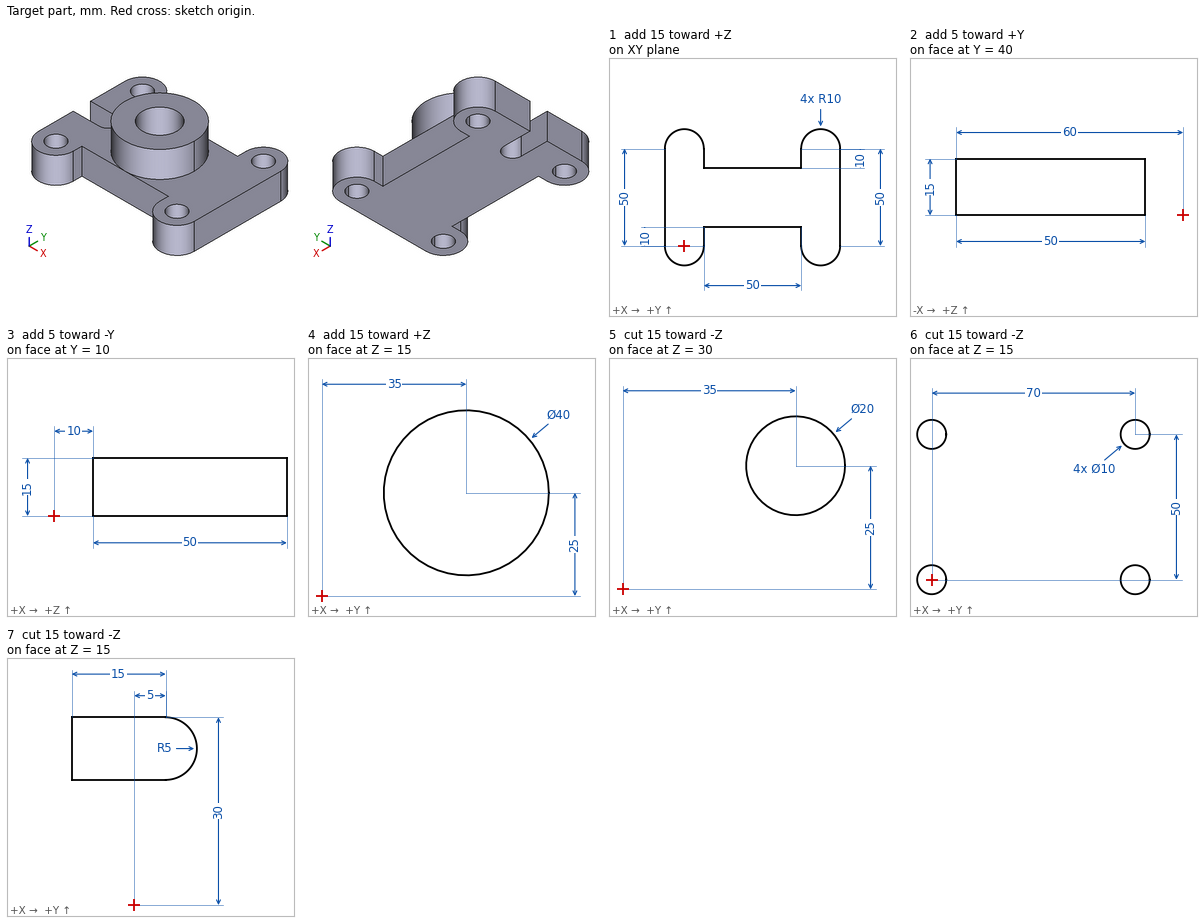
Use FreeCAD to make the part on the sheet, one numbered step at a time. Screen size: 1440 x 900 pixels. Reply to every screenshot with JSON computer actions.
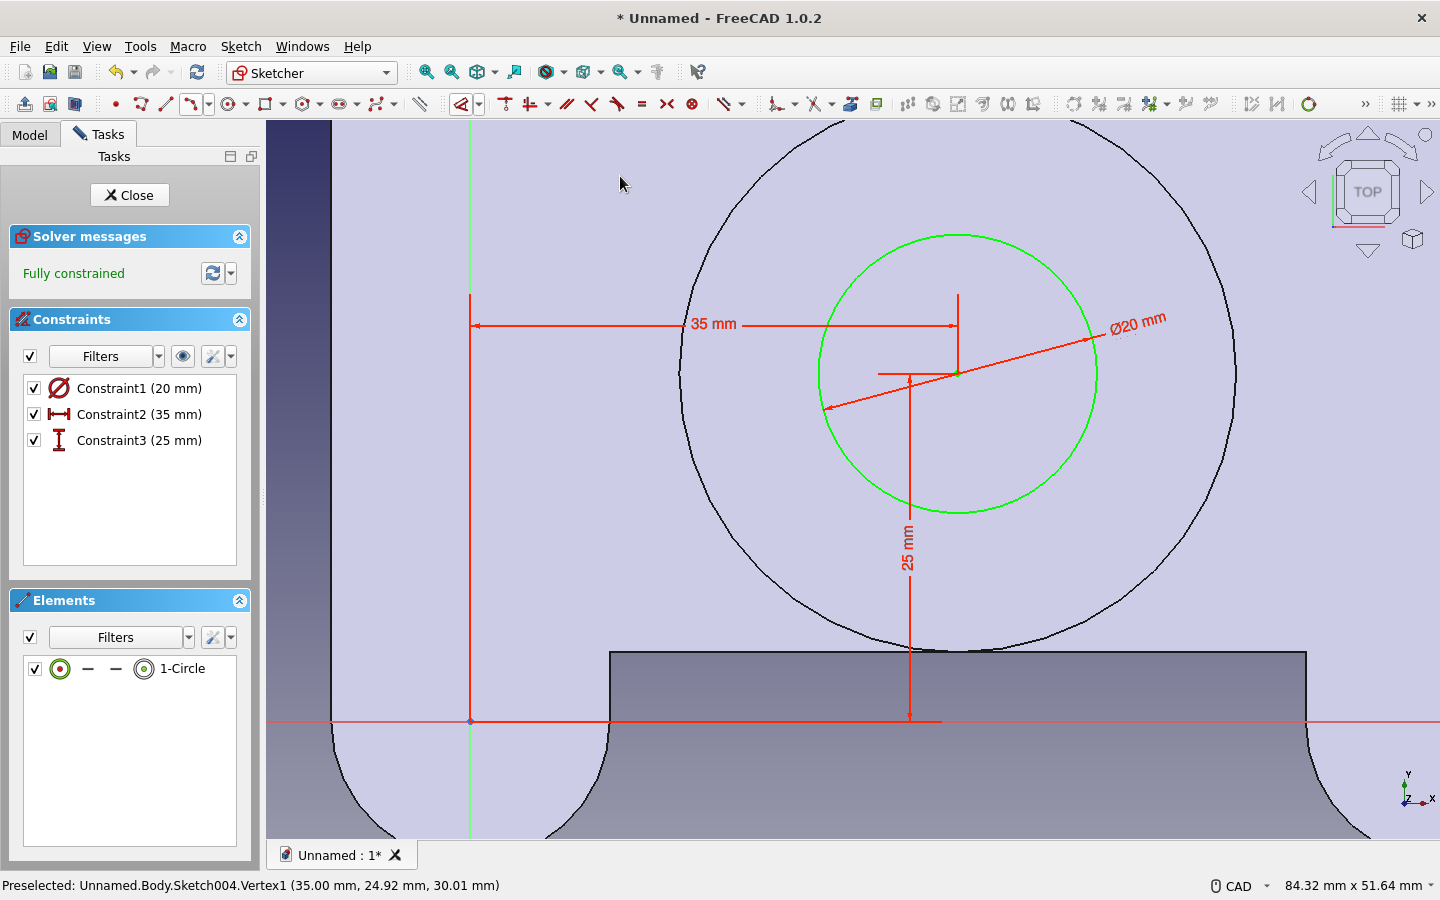
{"action": "left_click", "coordinate": [130, 195]}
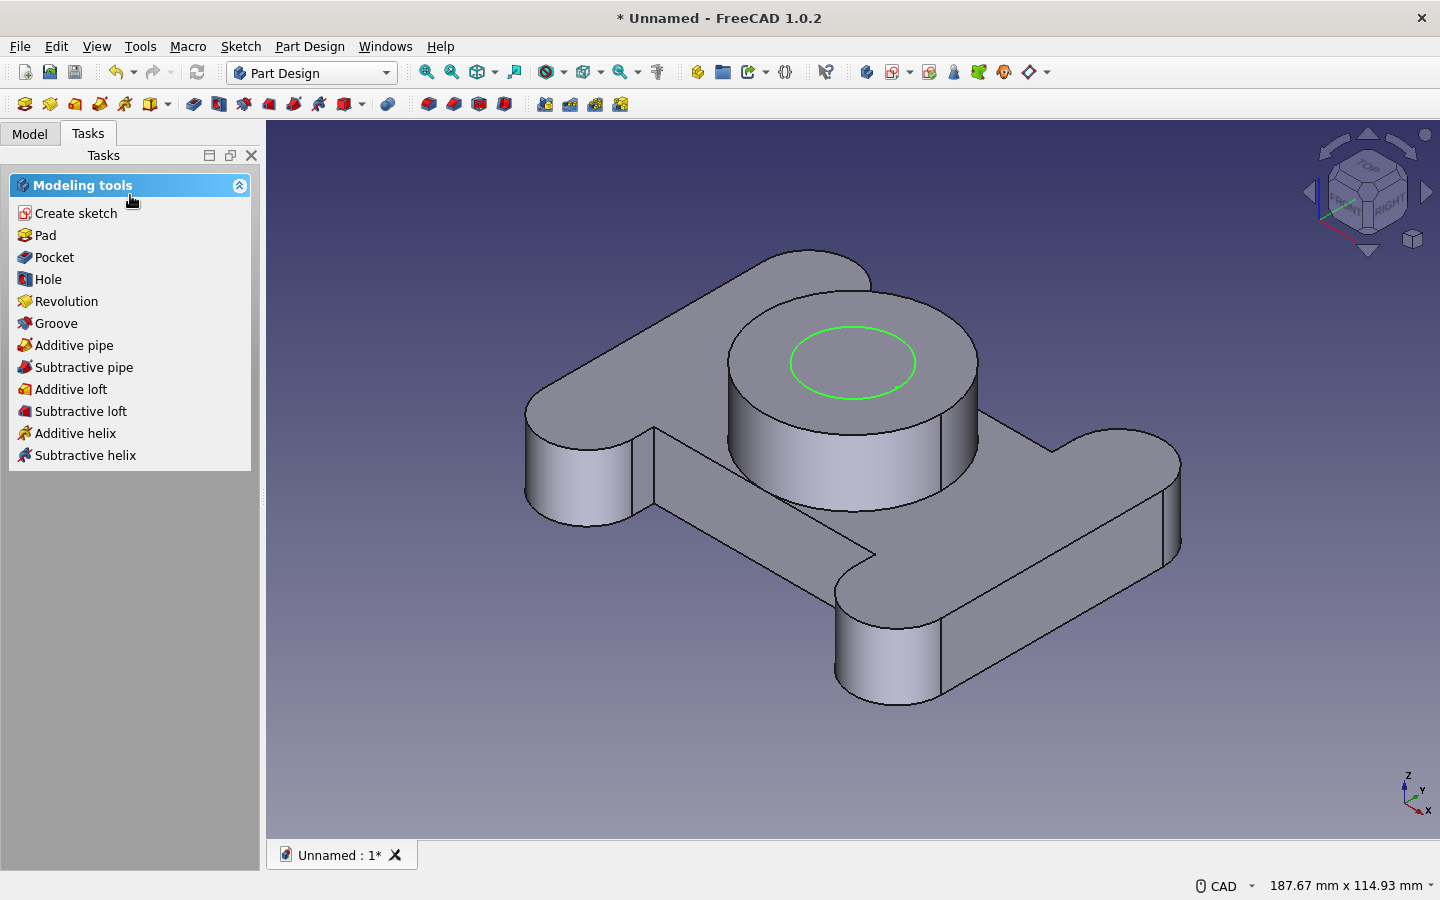
{"action": "left_click", "coordinate": [194, 104]}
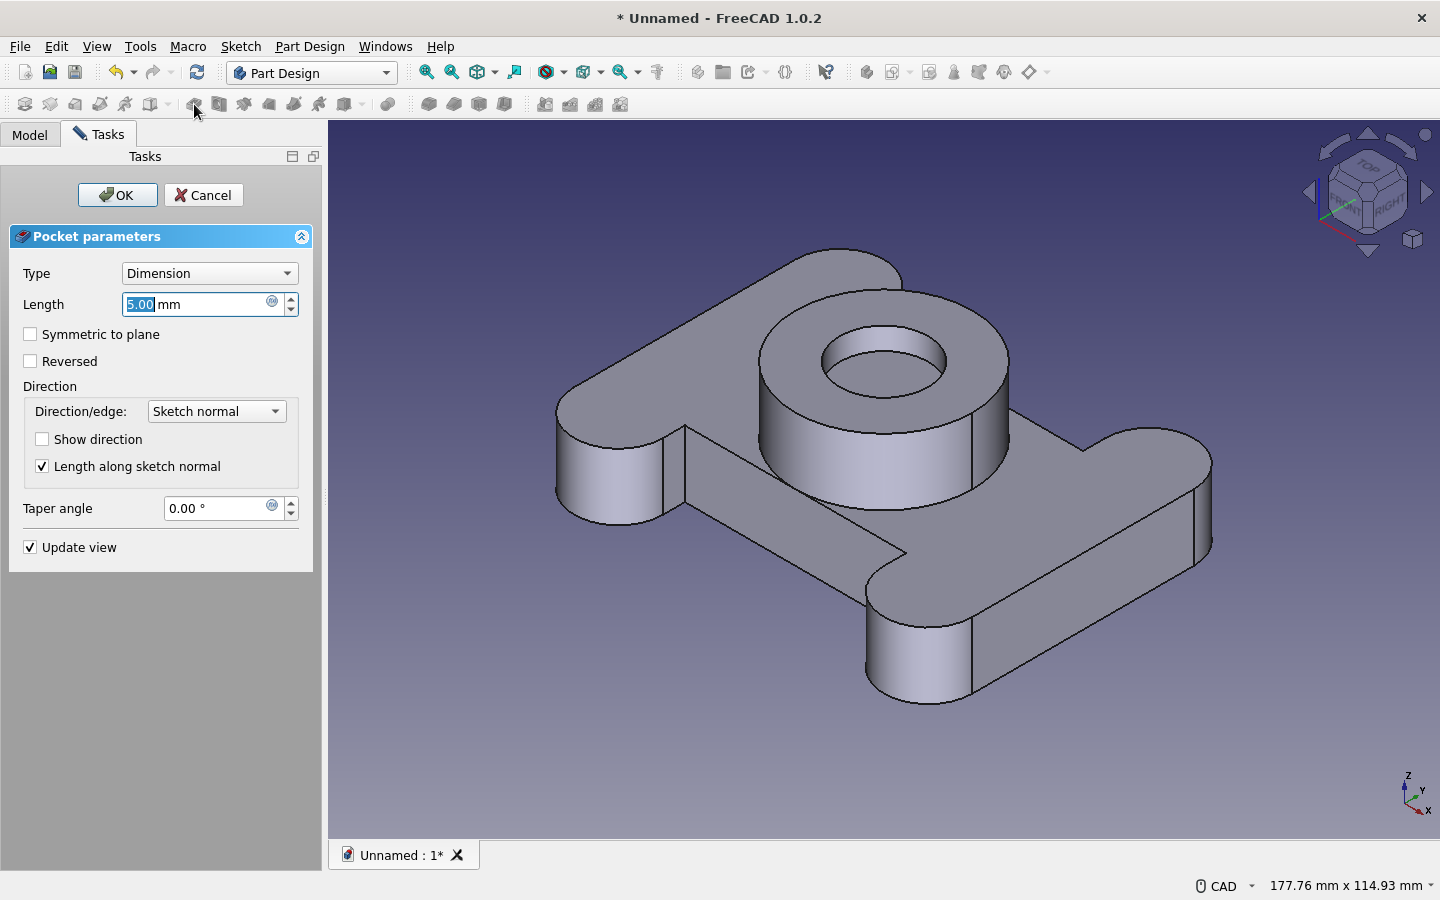
{"action": "type", "text": "15"}
{"action": "key", "text": "Tab"}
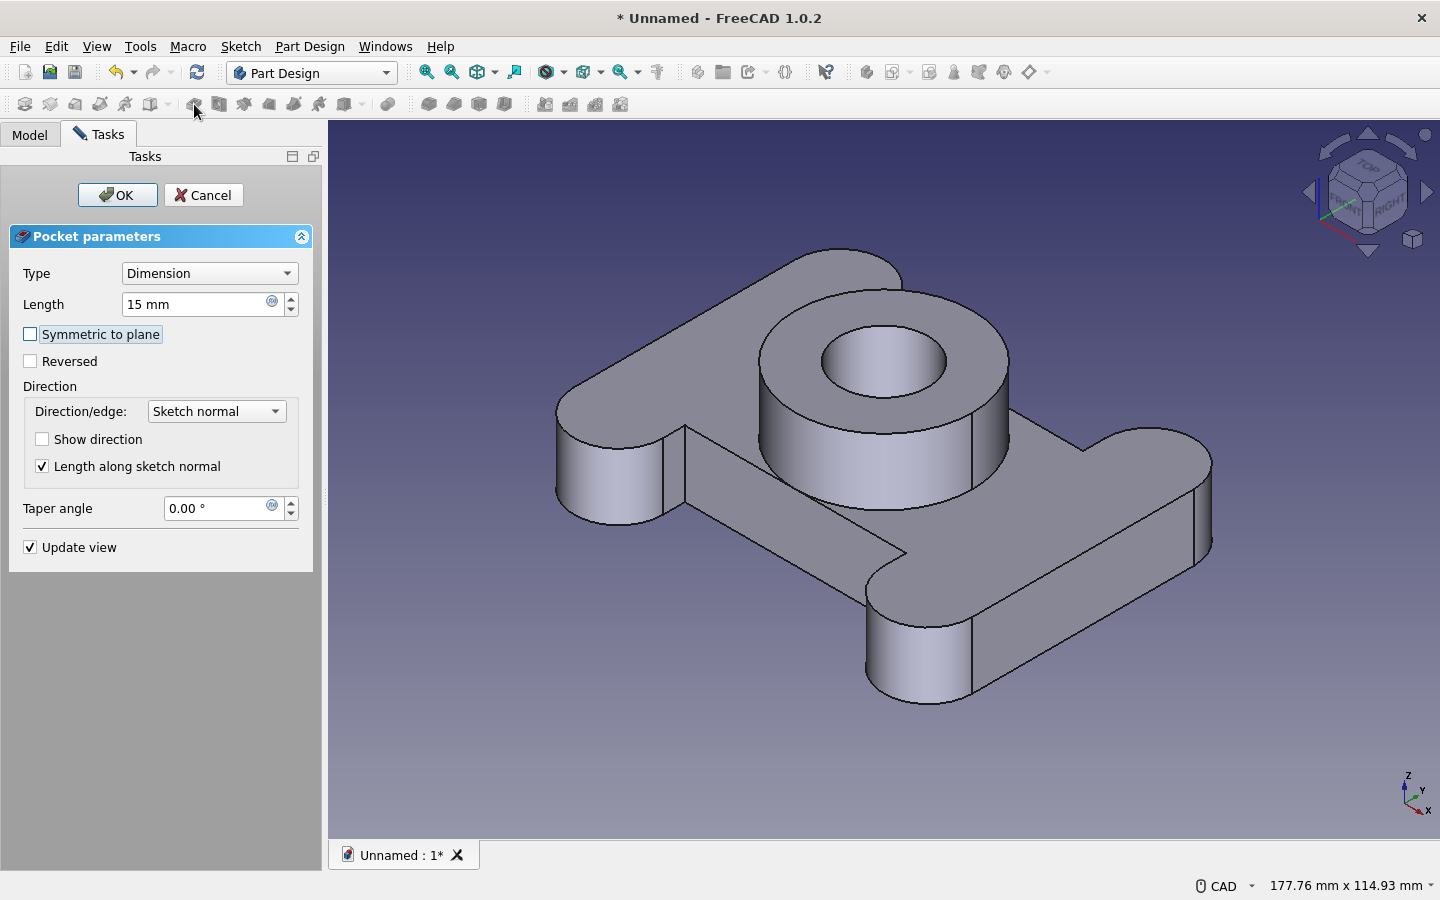
{"action": "left_click", "coordinate": [118, 195]}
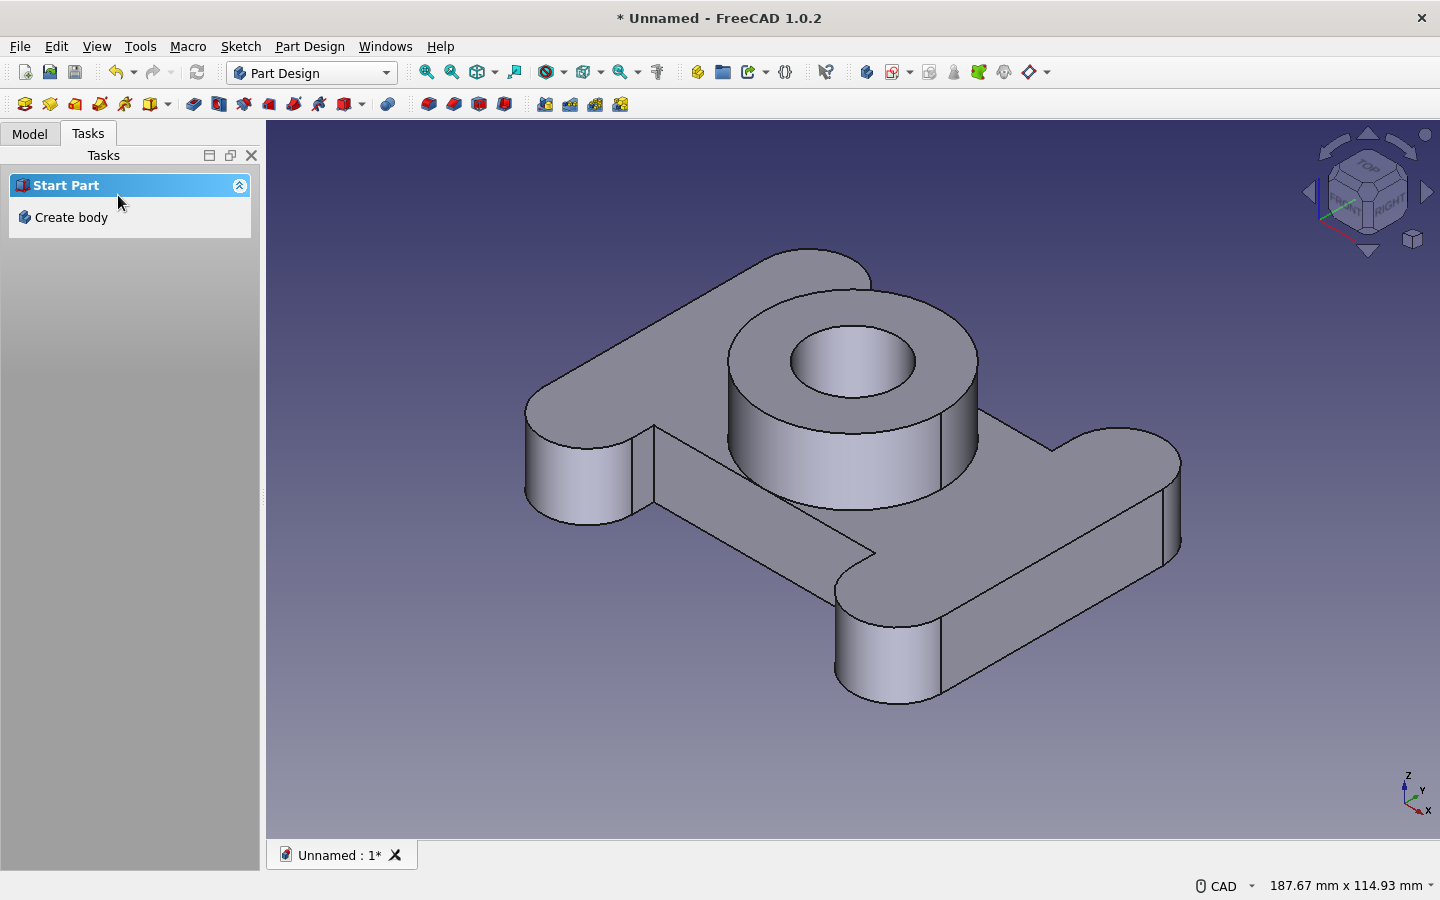
{"action": "left_click", "coordinate": [681, 389]}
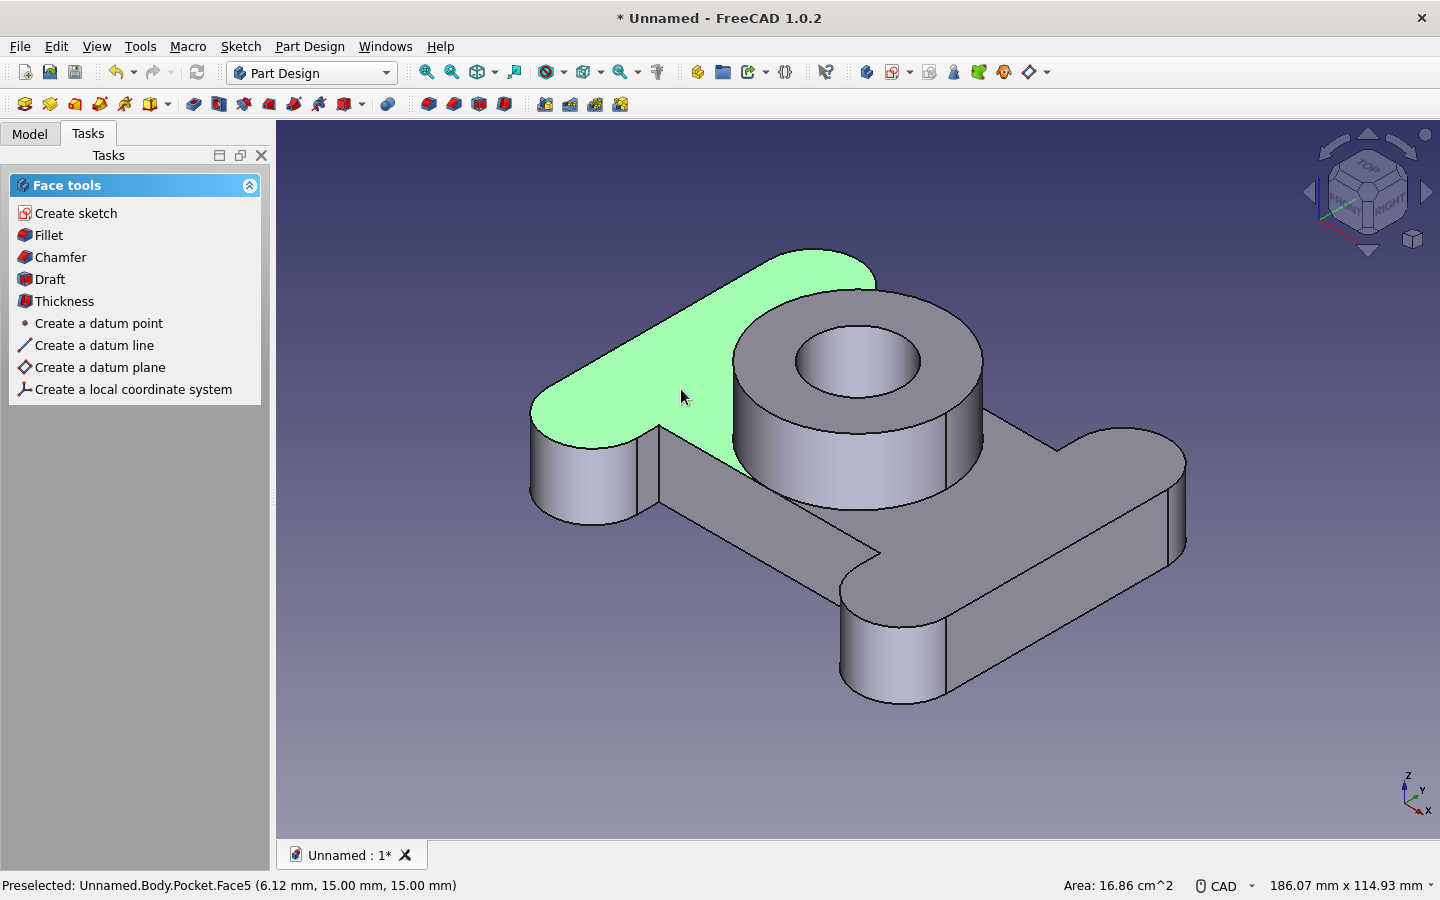
{"action": "left_click", "coordinate": [892, 72]}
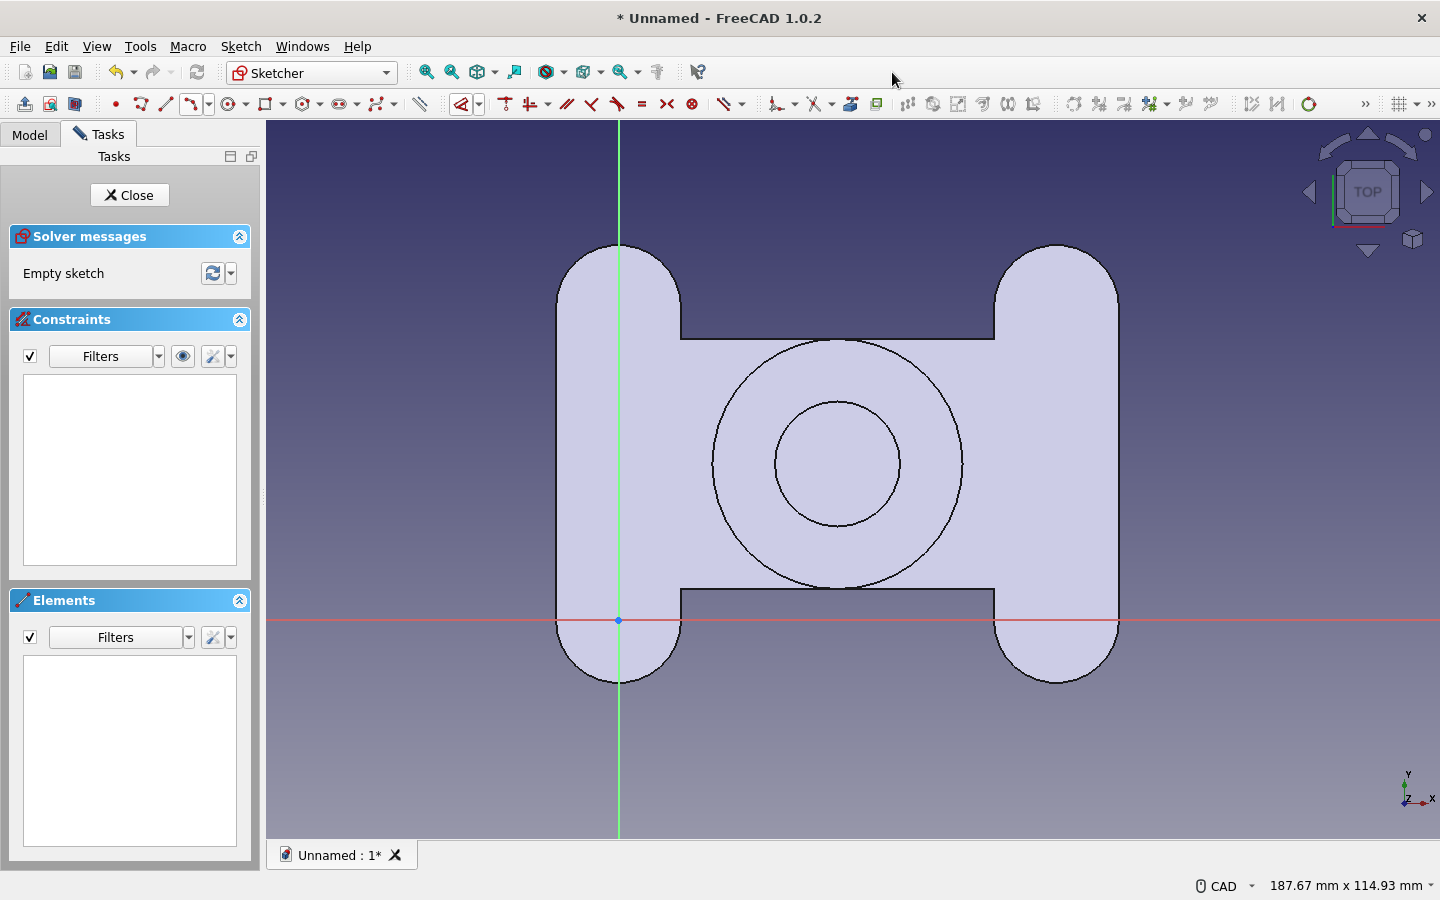
{"action": "left_click", "coordinate": [75, 104]}